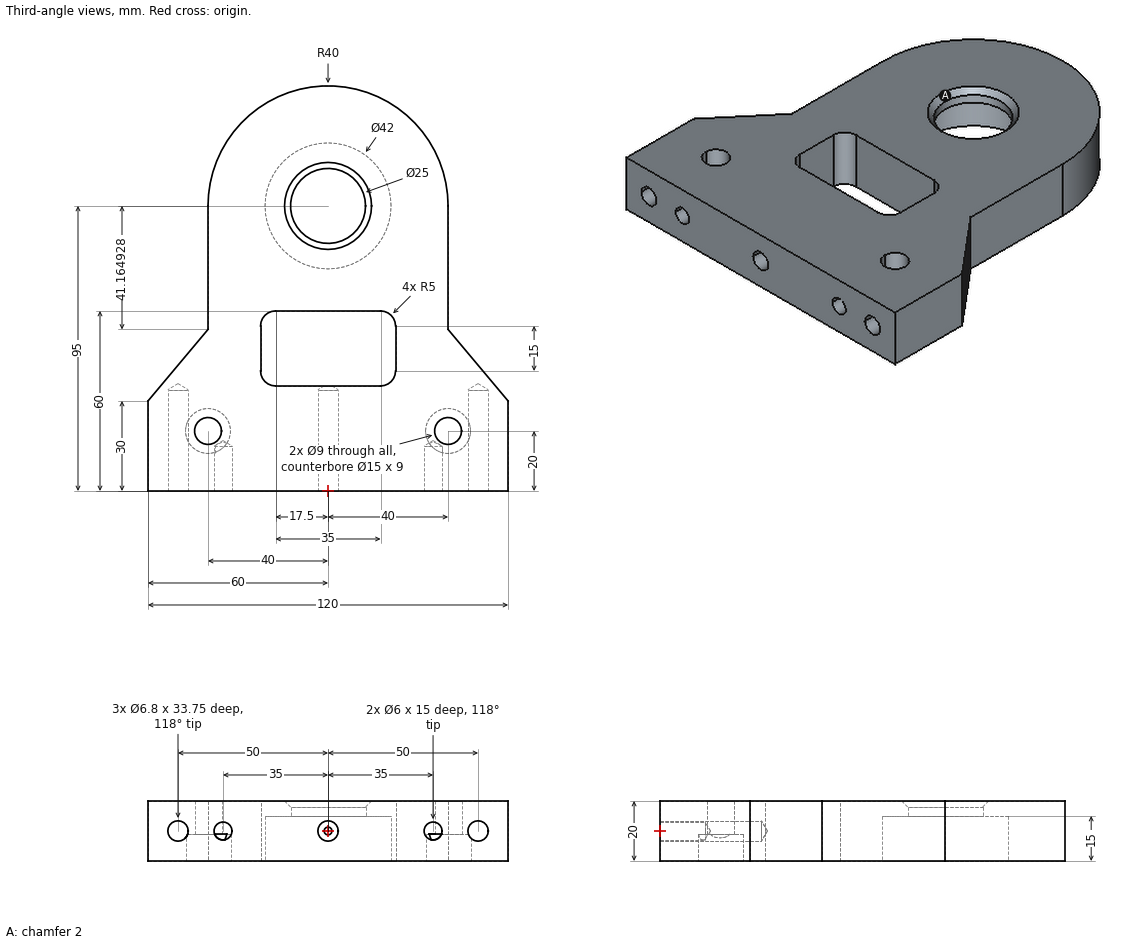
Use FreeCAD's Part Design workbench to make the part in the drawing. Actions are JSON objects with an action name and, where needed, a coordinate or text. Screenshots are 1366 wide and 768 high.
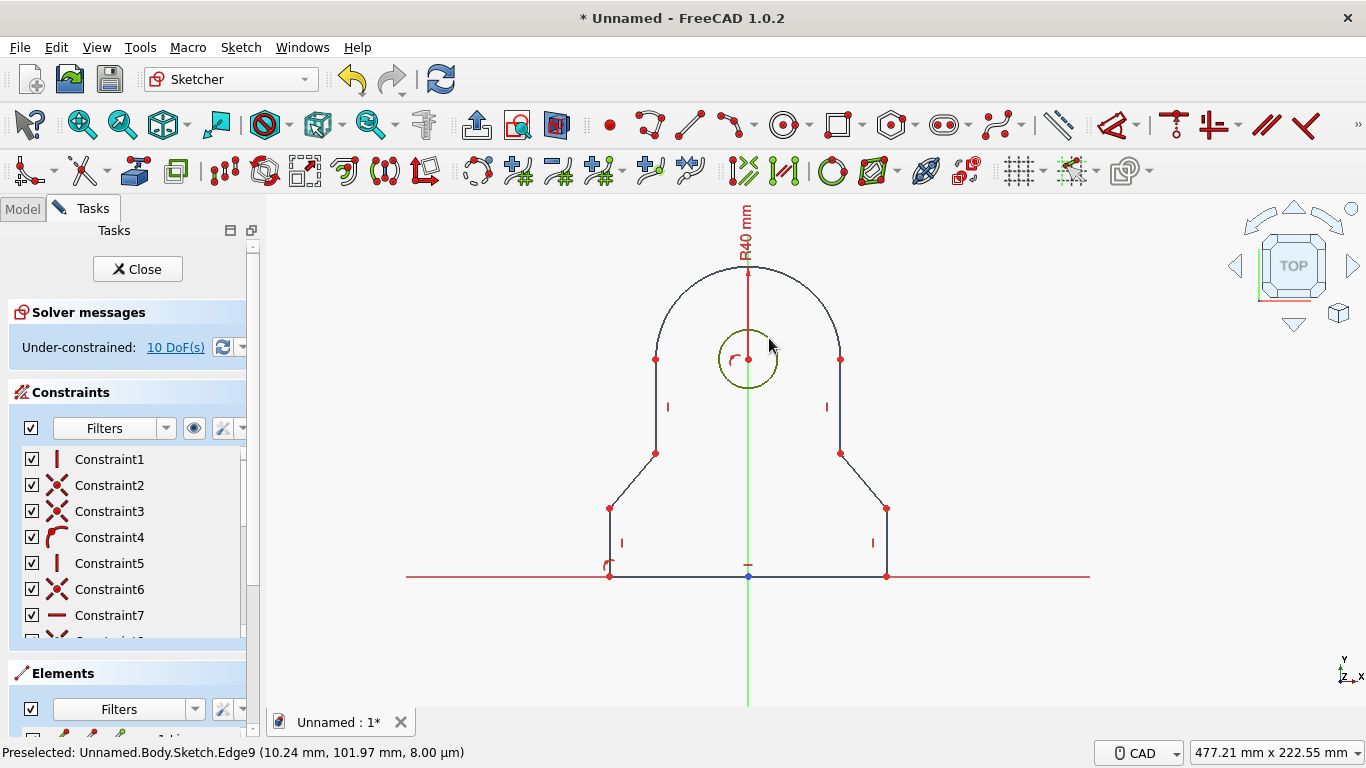
{"action": "left_click", "coordinate": [1138, 126]}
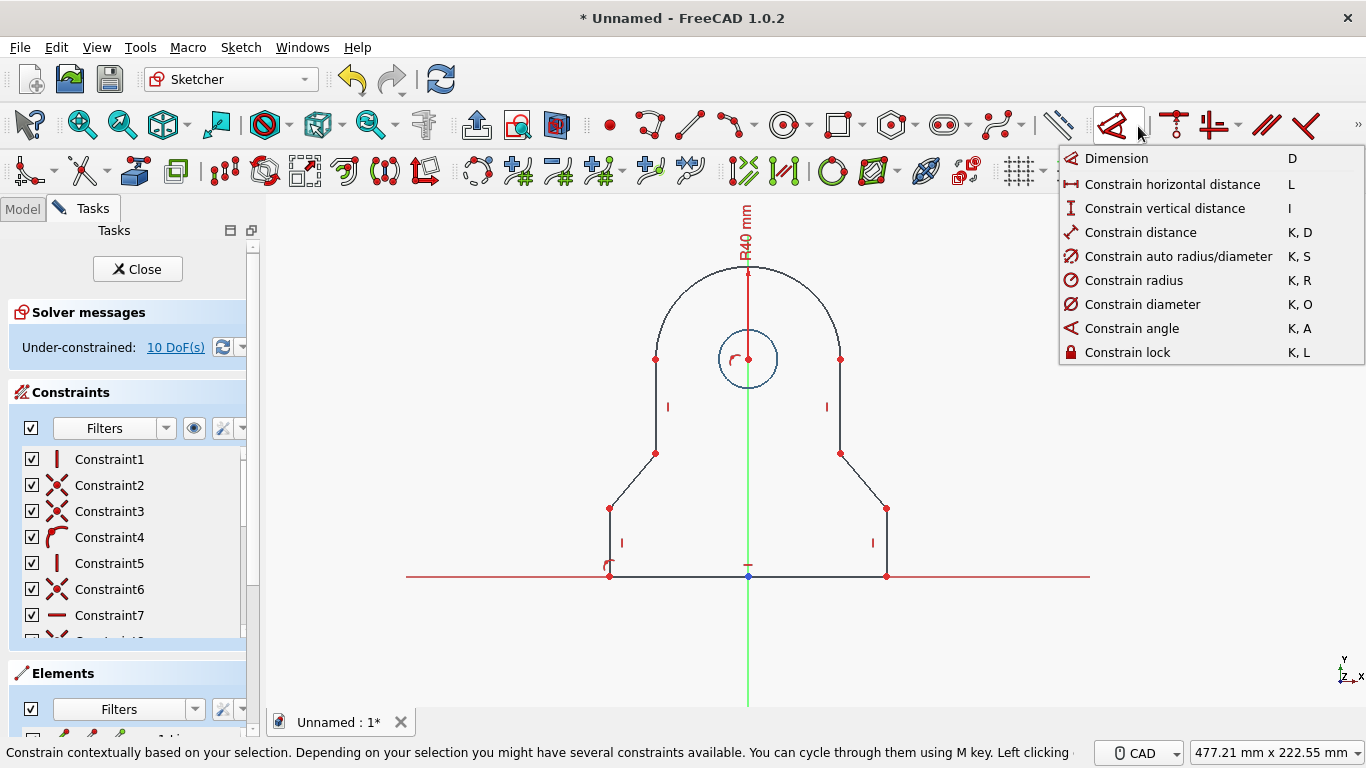
{"action": "left_click", "coordinate": [1212, 304]}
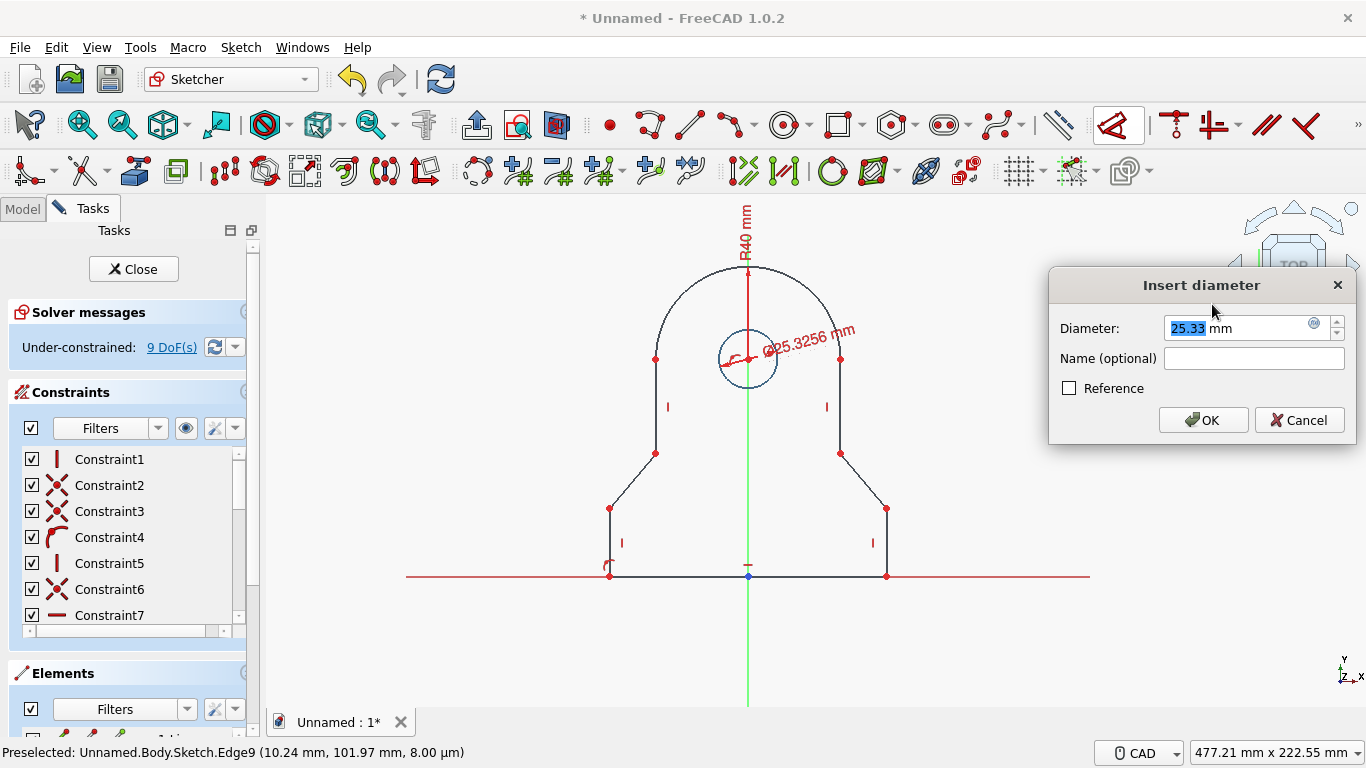
{"action": "type", "text": "25"}
{"action": "key", "text": "Return"}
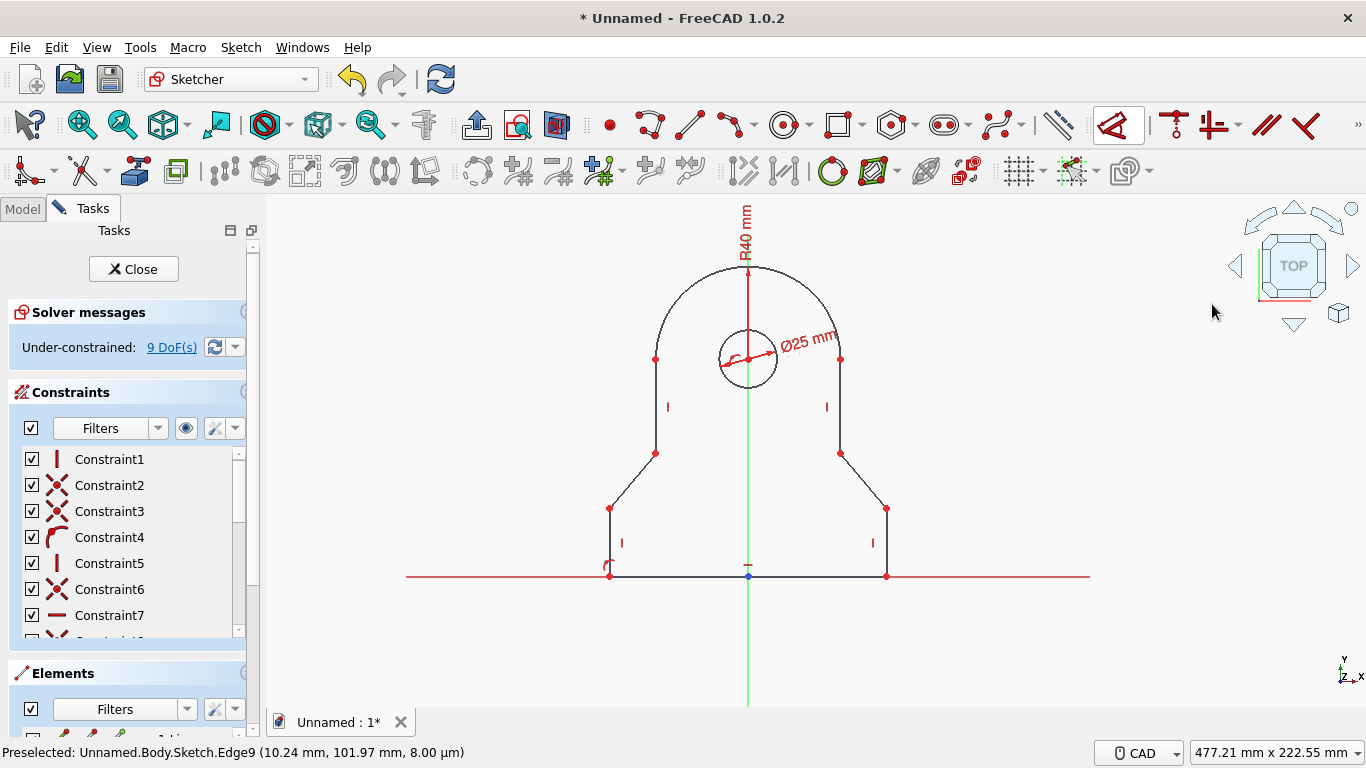
{"action": "left_click", "coordinate": [610, 529]}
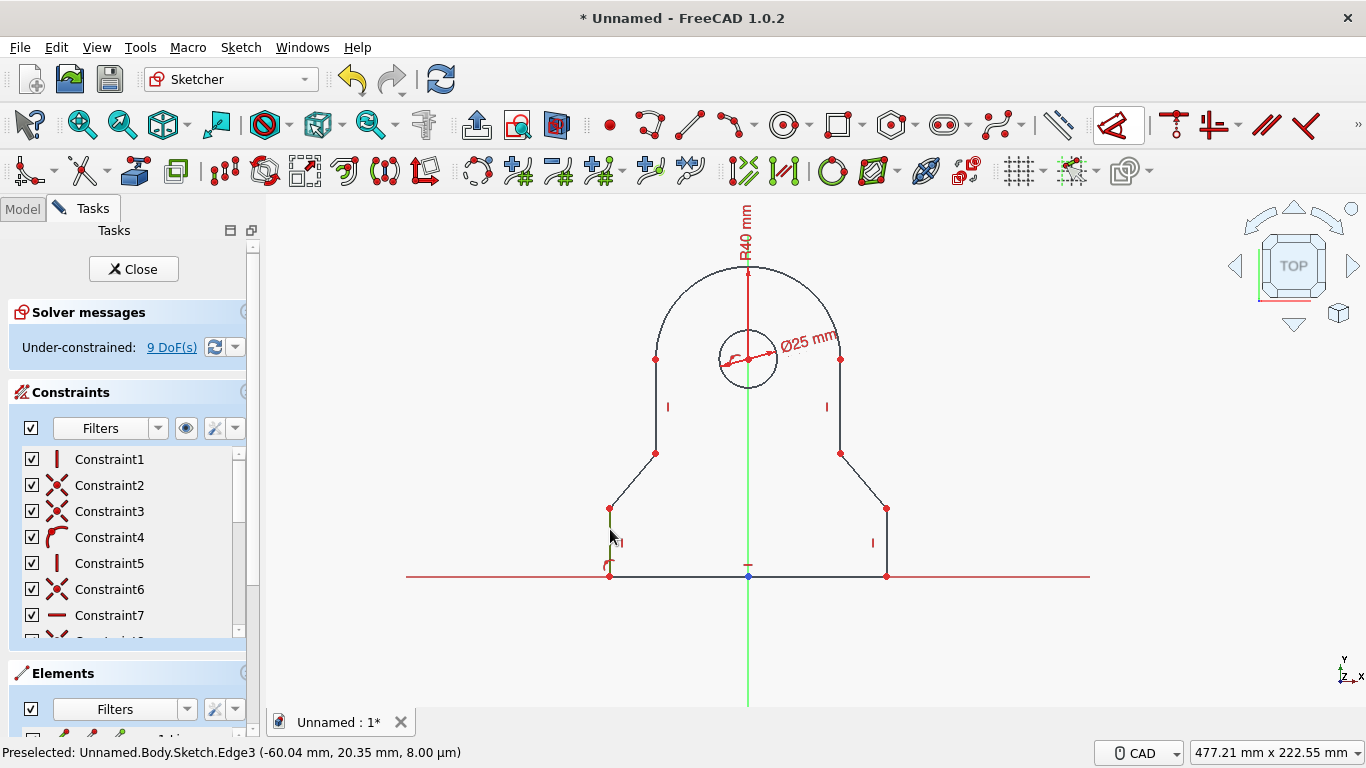
{"action": "left_click", "coordinate": [1138, 126]}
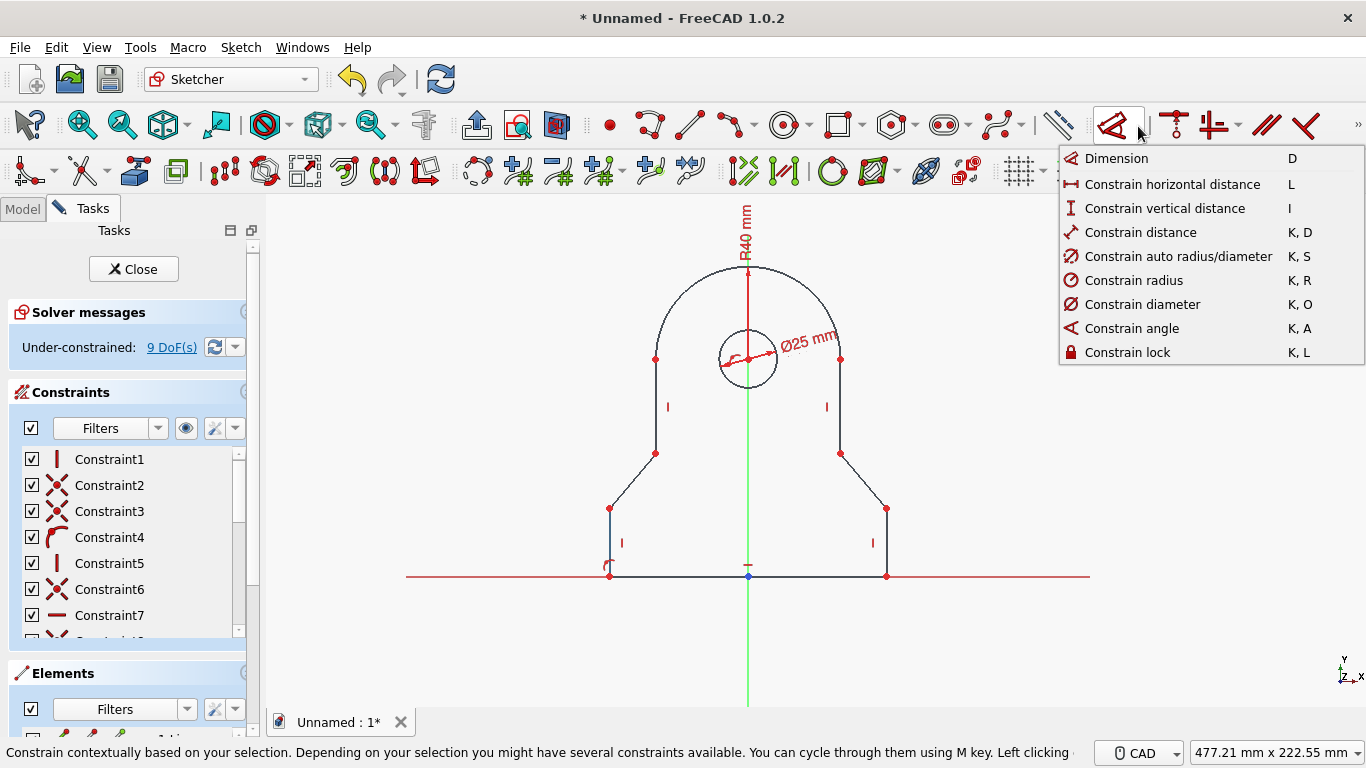
{"action": "left_click", "coordinate": [1212, 208]}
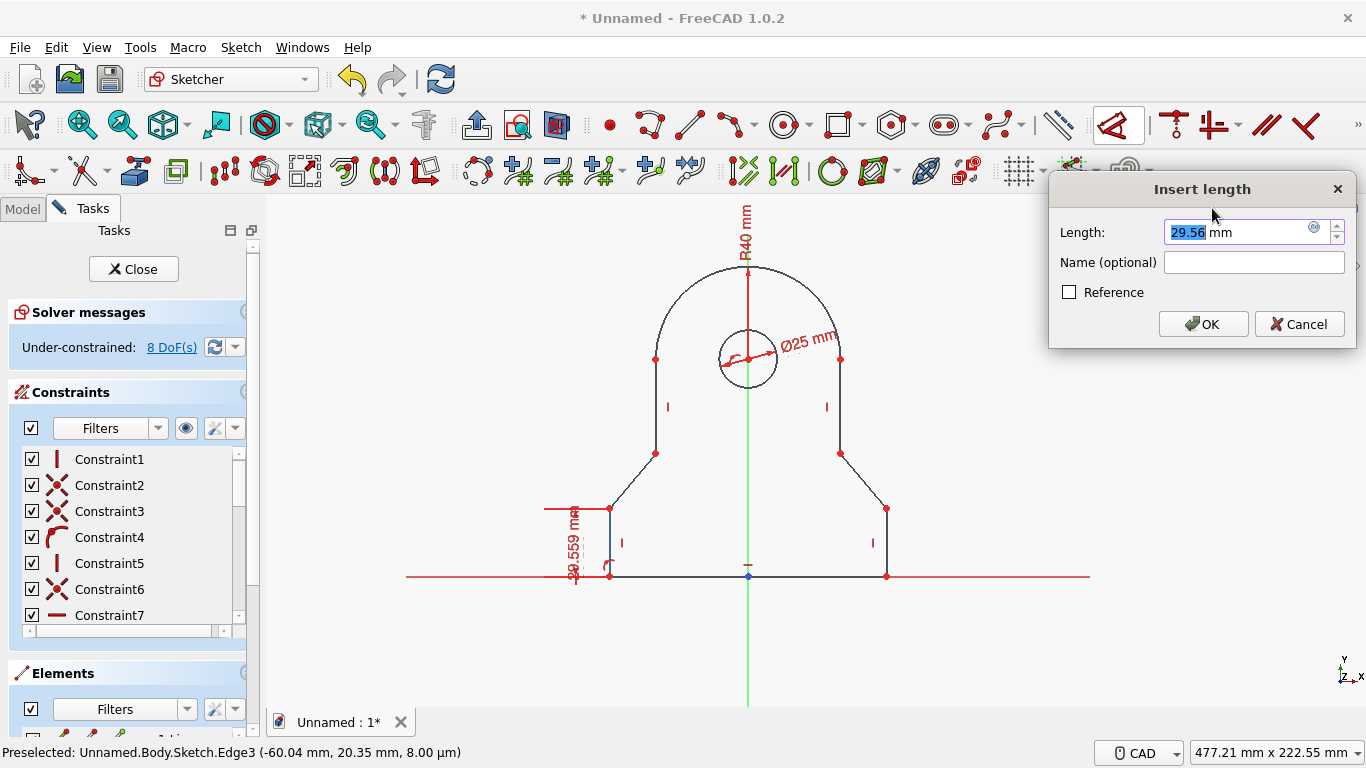
{"action": "type", "text": "30"}
{"action": "key", "text": "Return"}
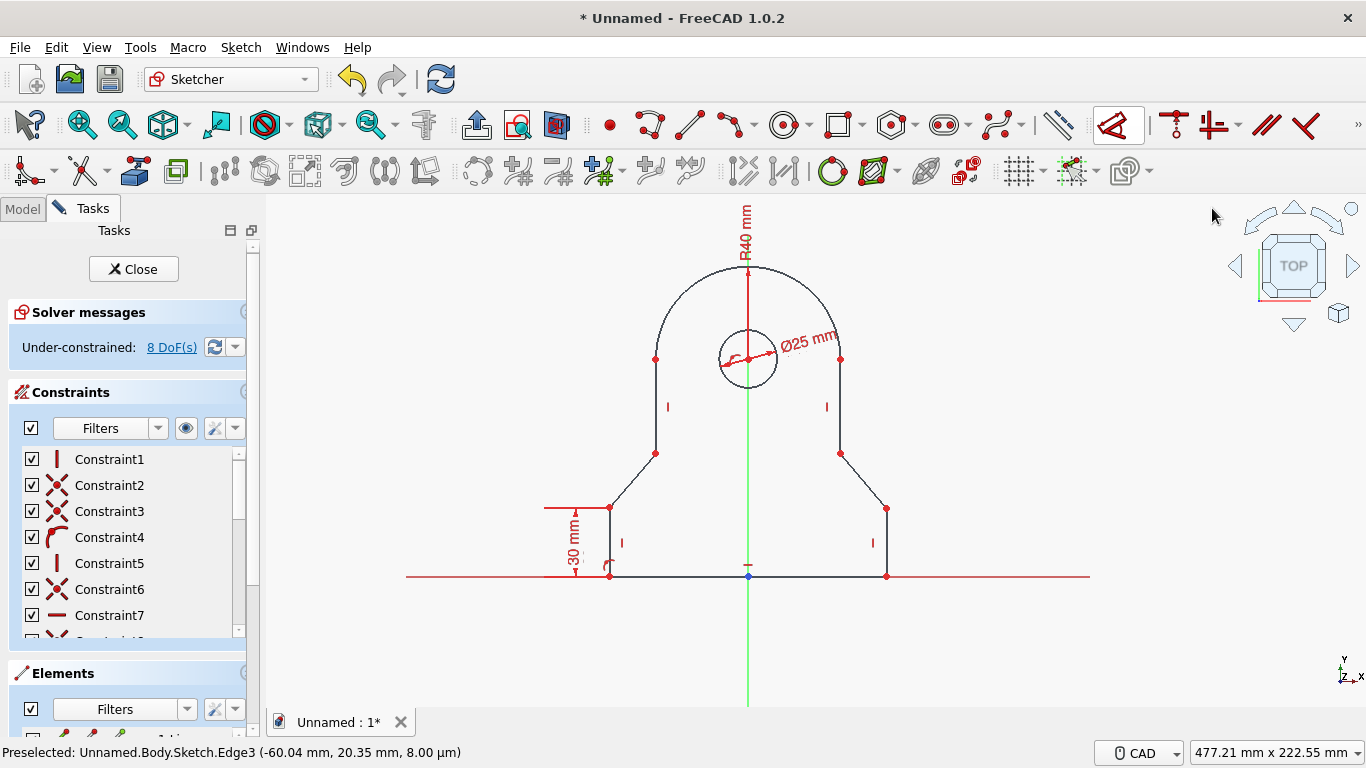
{"action": "left_click", "coordinate": [887, 556]}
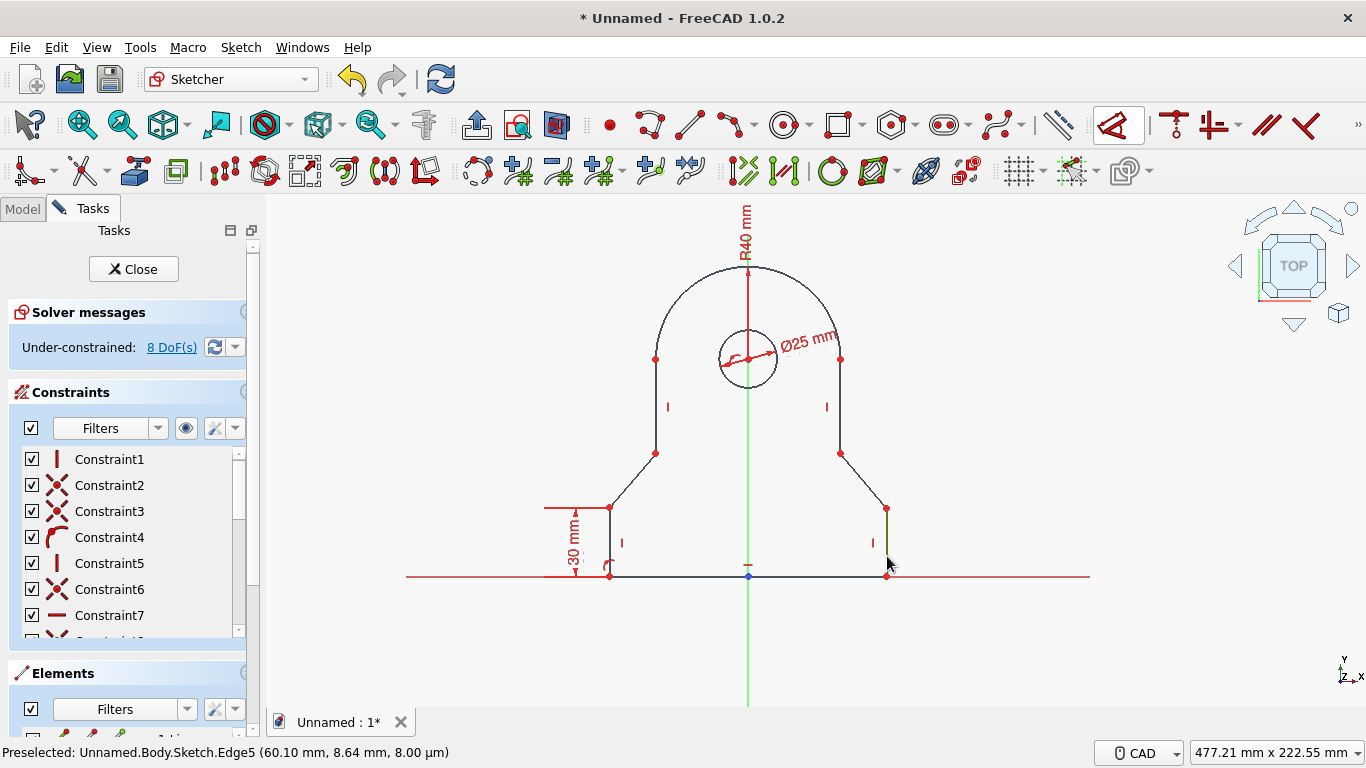
{"action": "key", "text": "i"}